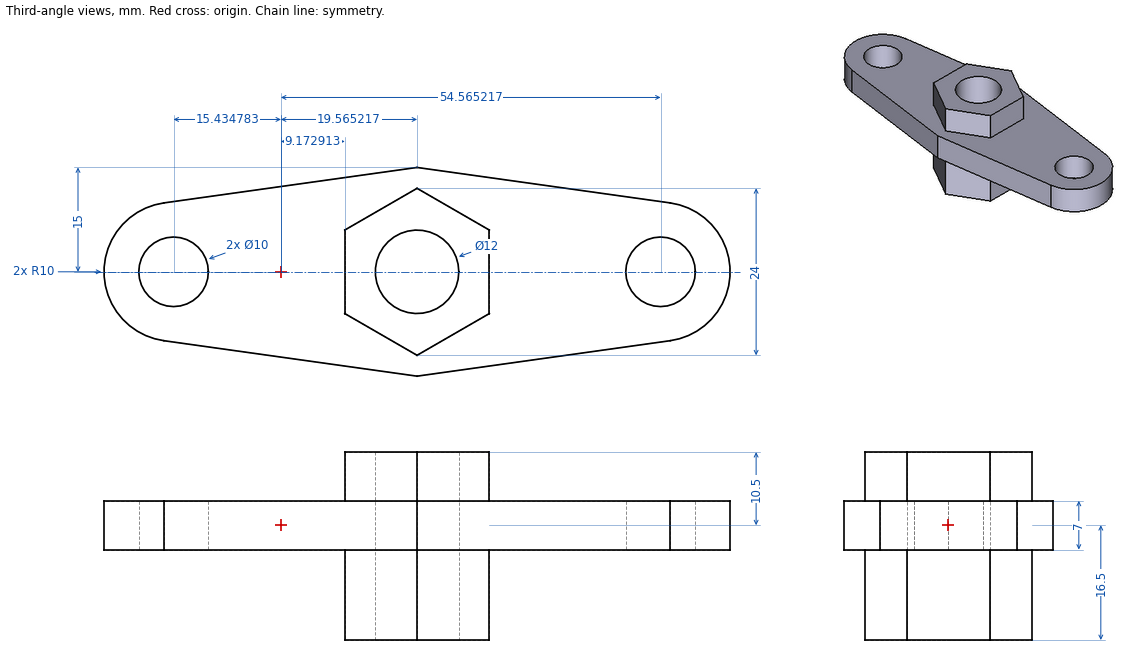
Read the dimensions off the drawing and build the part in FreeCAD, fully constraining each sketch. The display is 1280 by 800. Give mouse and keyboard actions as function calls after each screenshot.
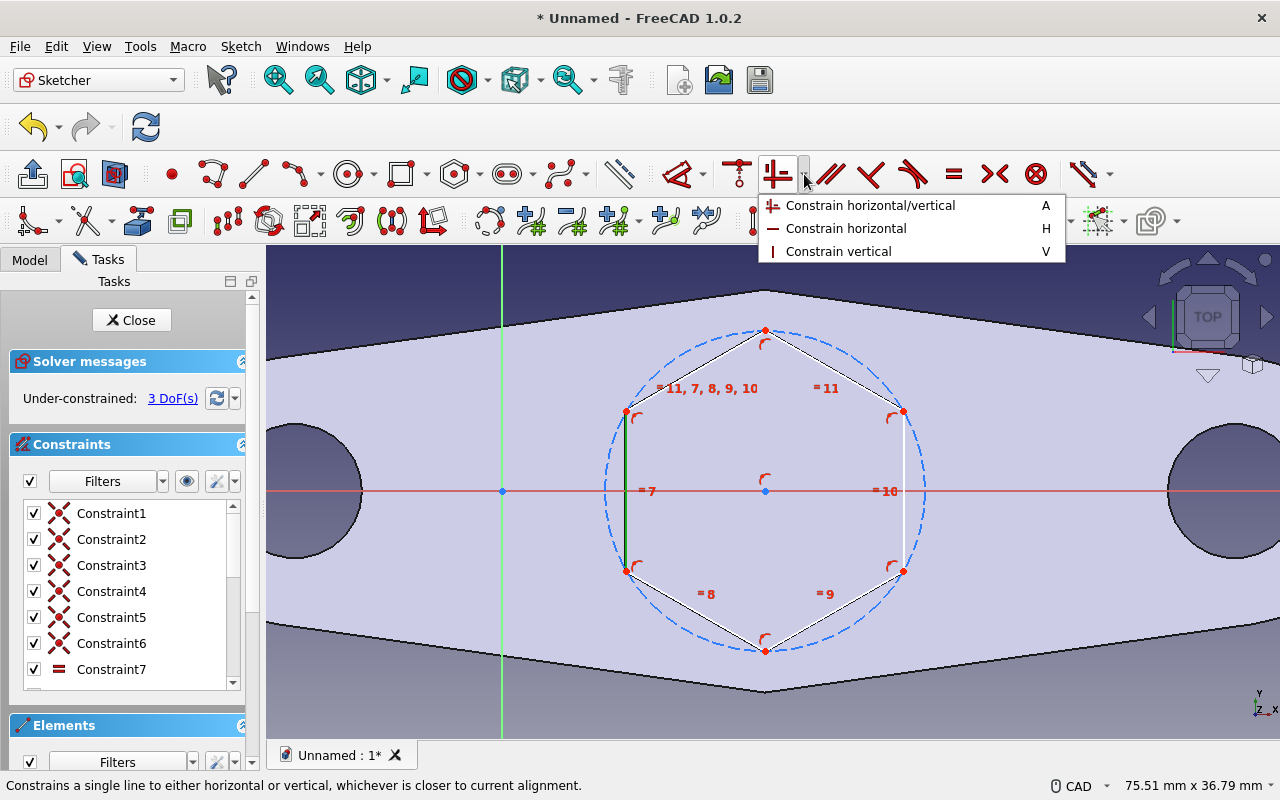
click(912, 252)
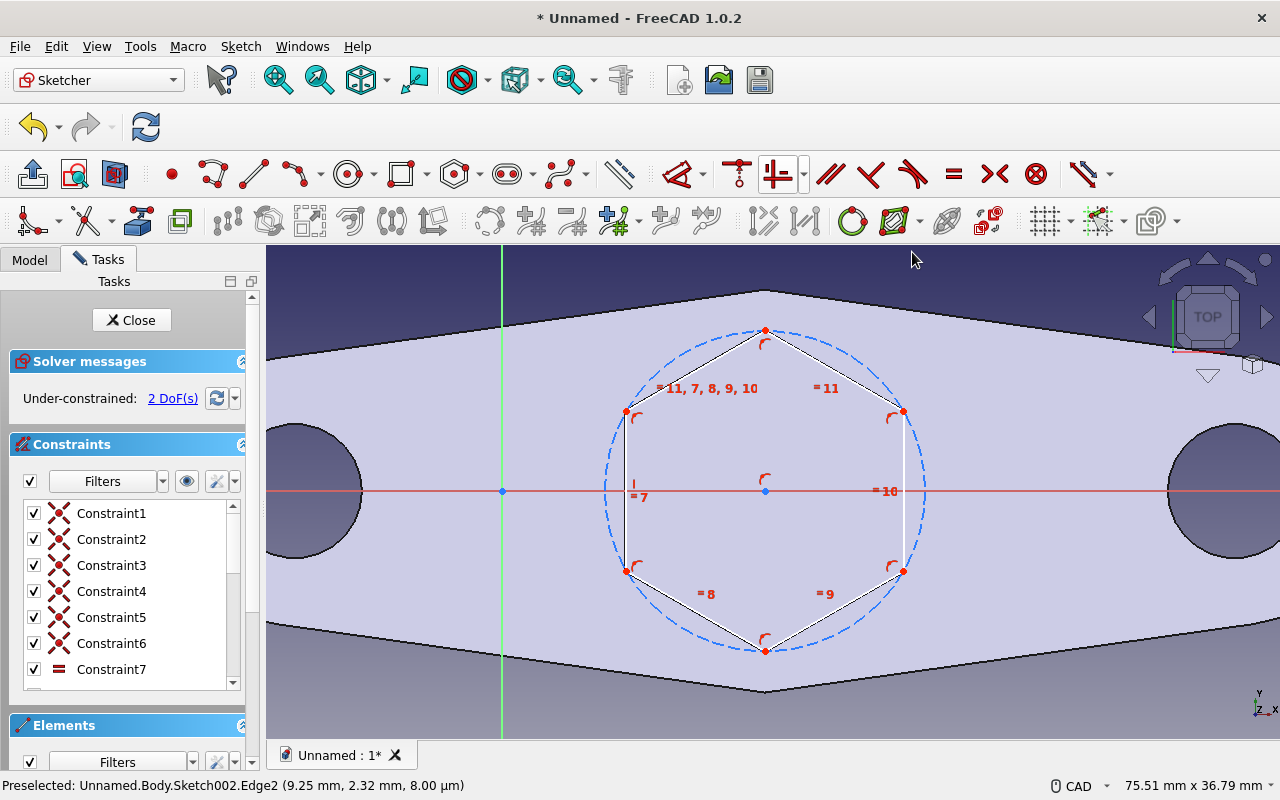
click(676, 174)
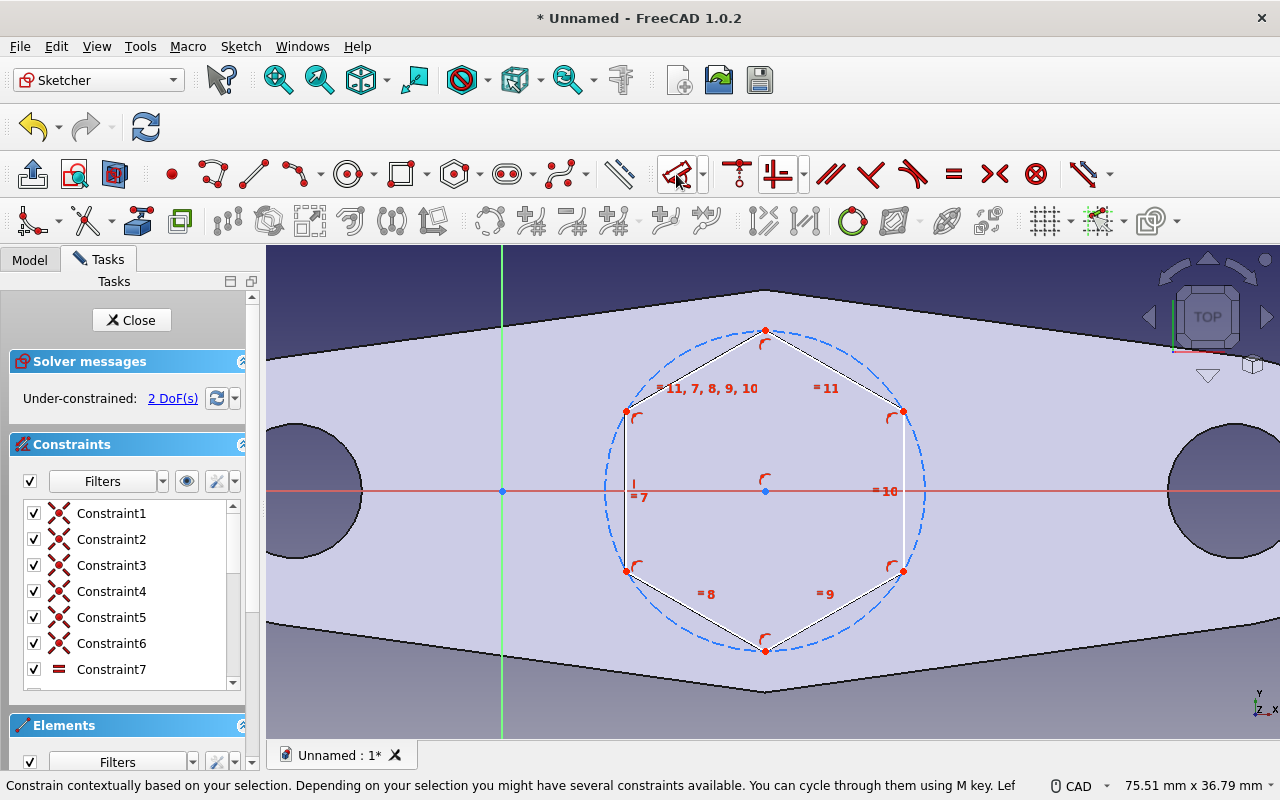
click(765, 651)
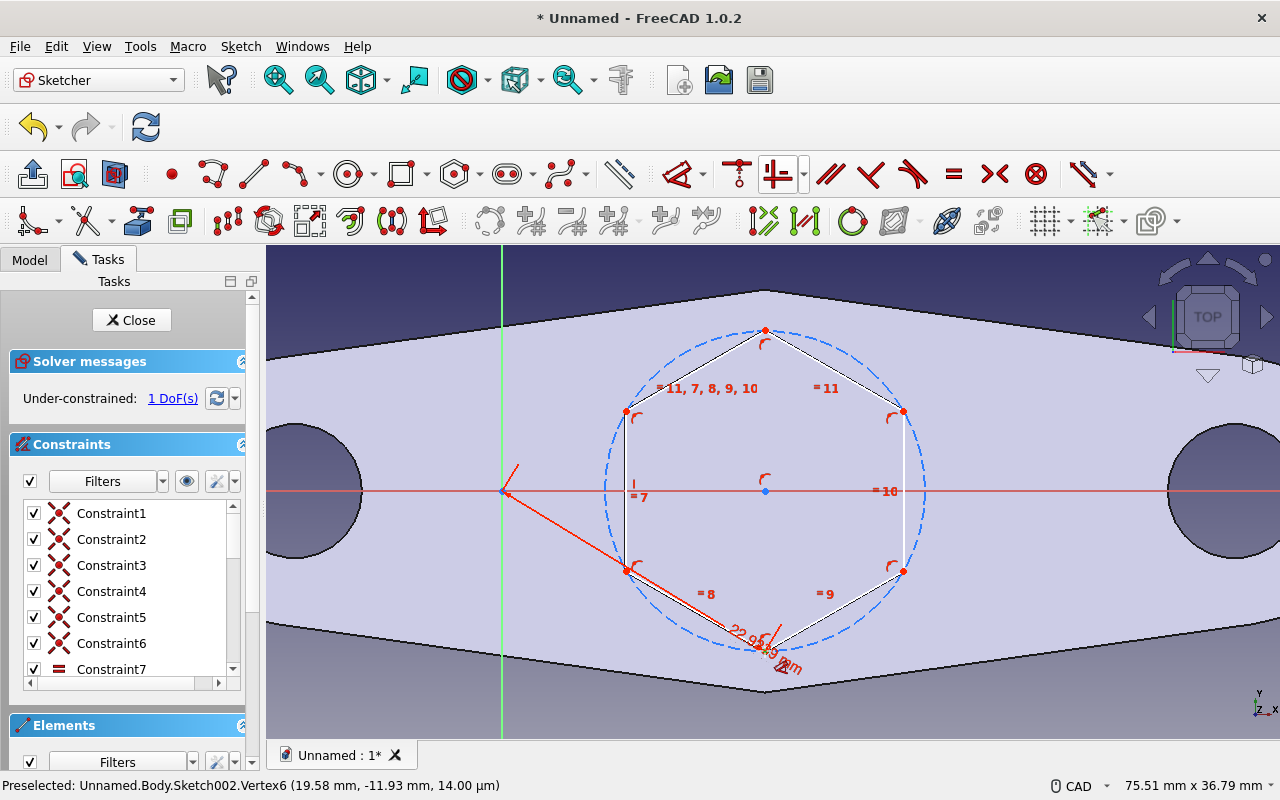
click(765, 331)
click(799, 417)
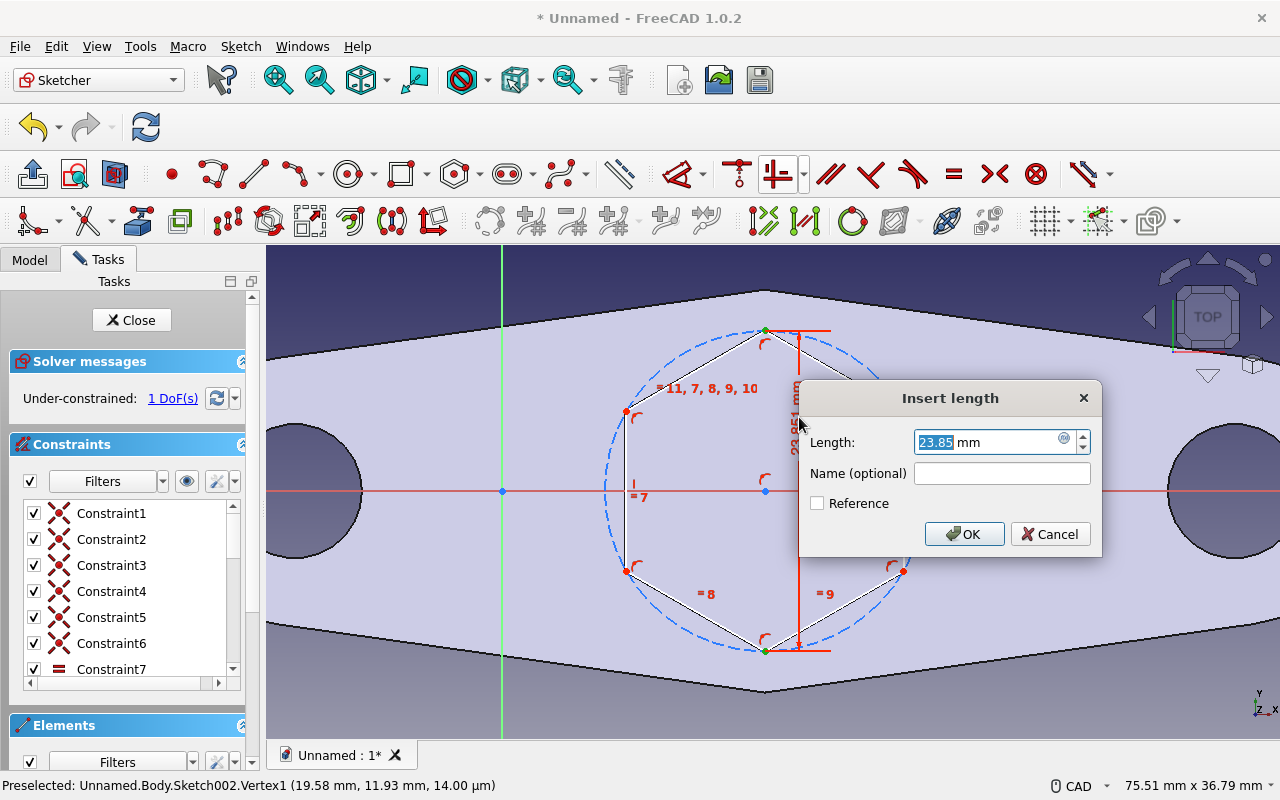
text(24)
key(Return)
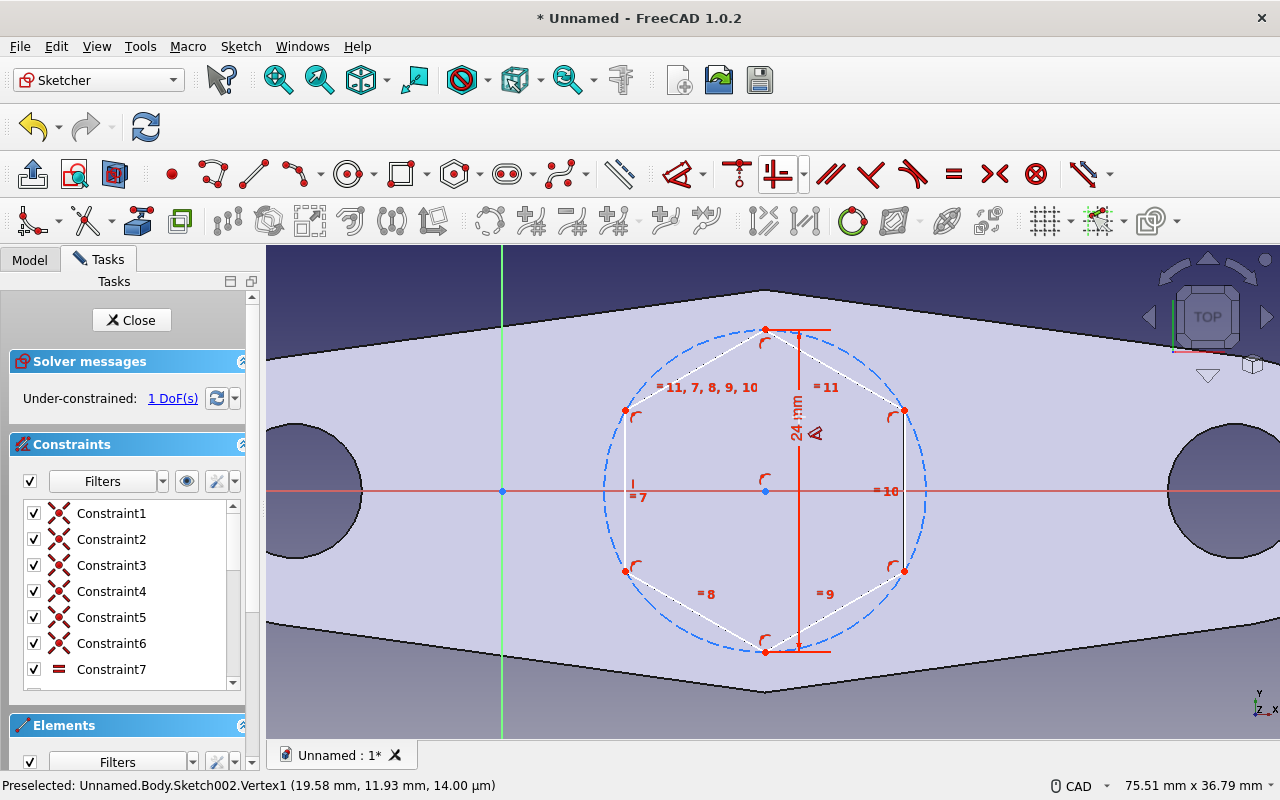
click(625, 411)
click(564, 377)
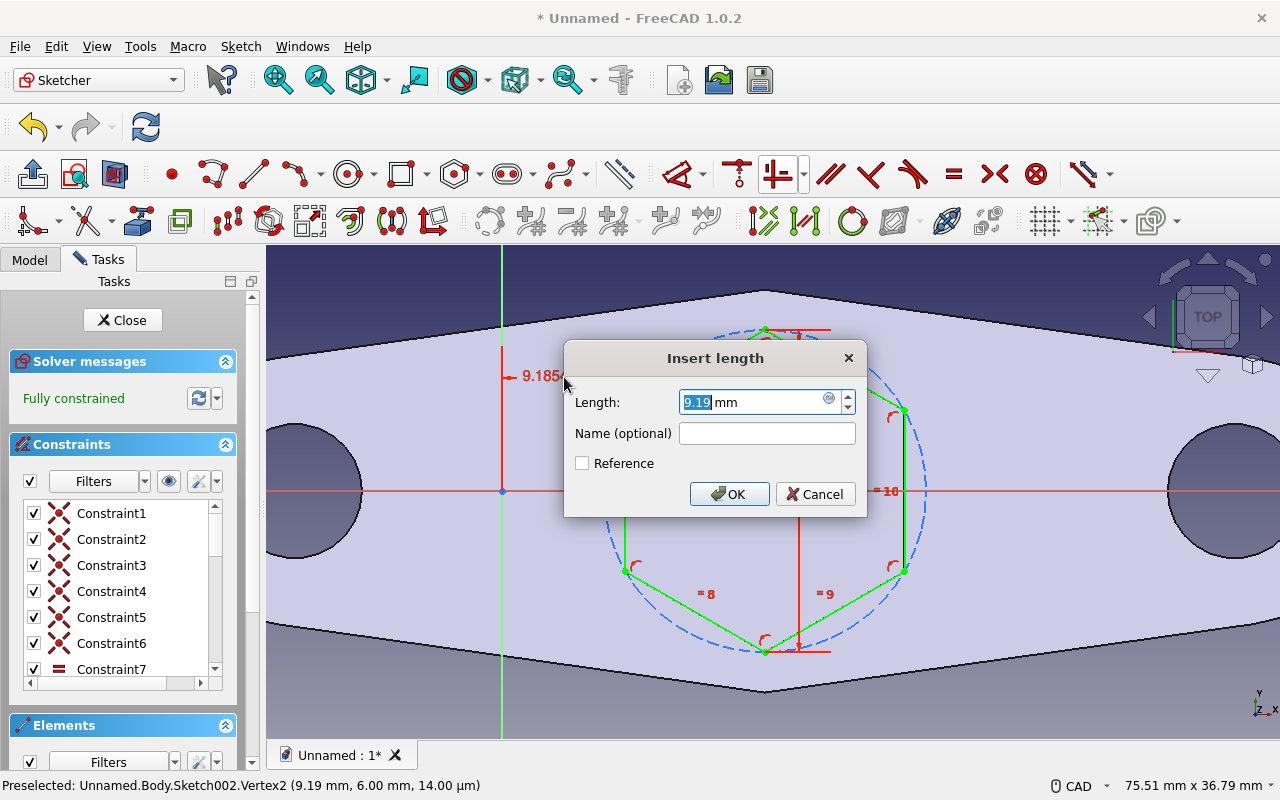
text(9.172913)
key(Return)
key(Escape)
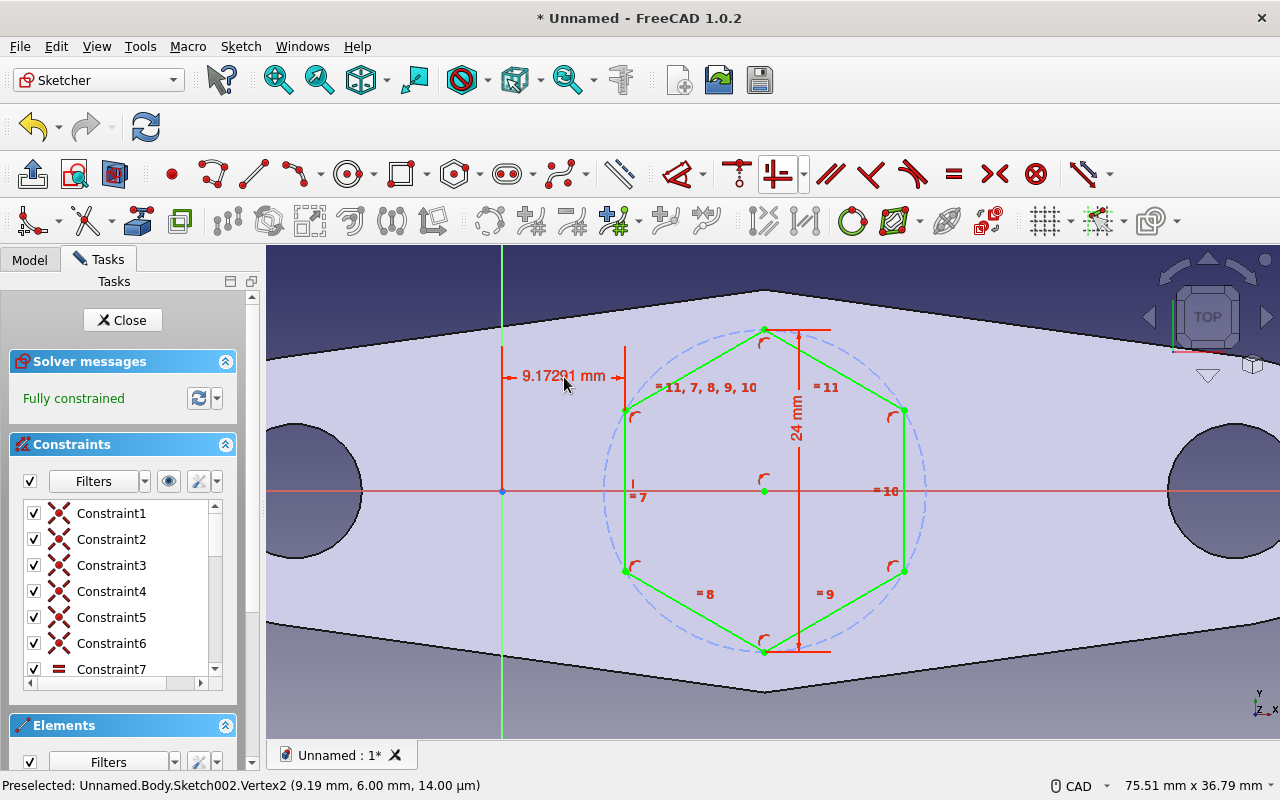
click(123, 320)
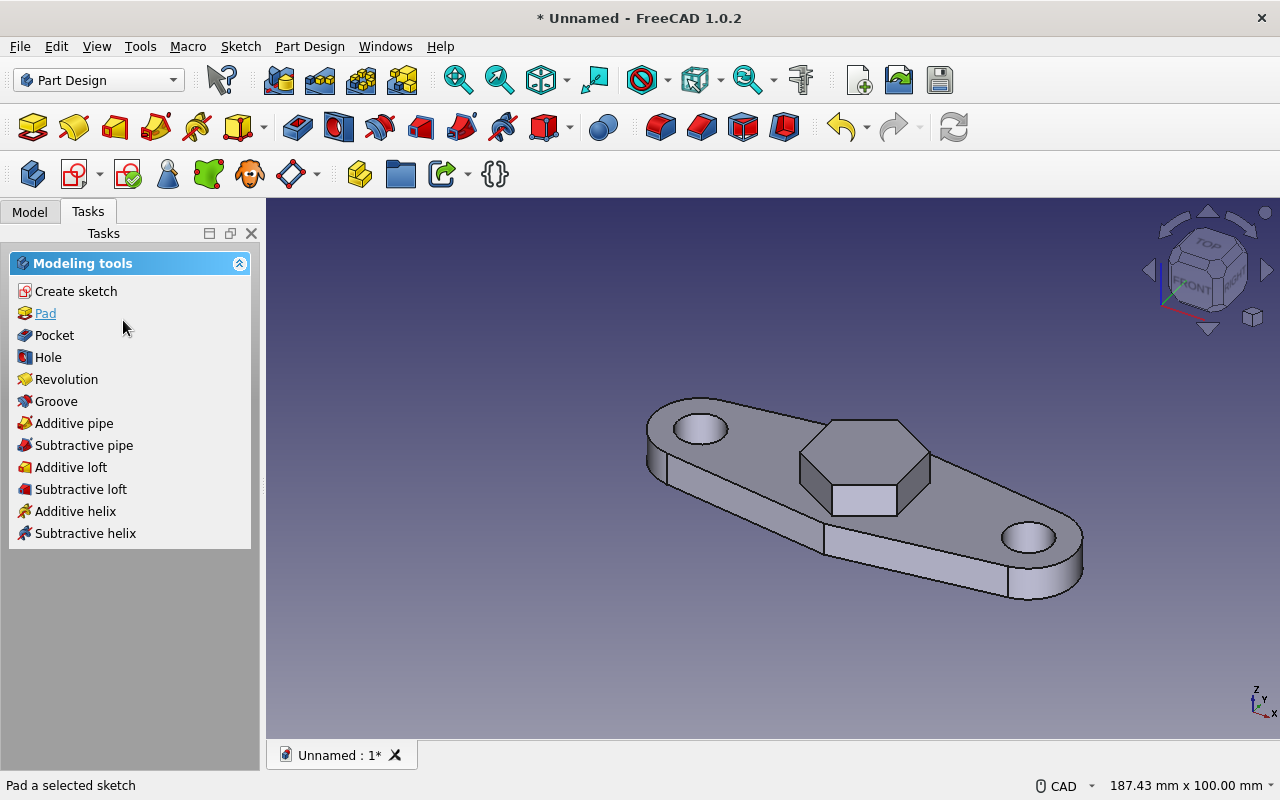
click(33, 128)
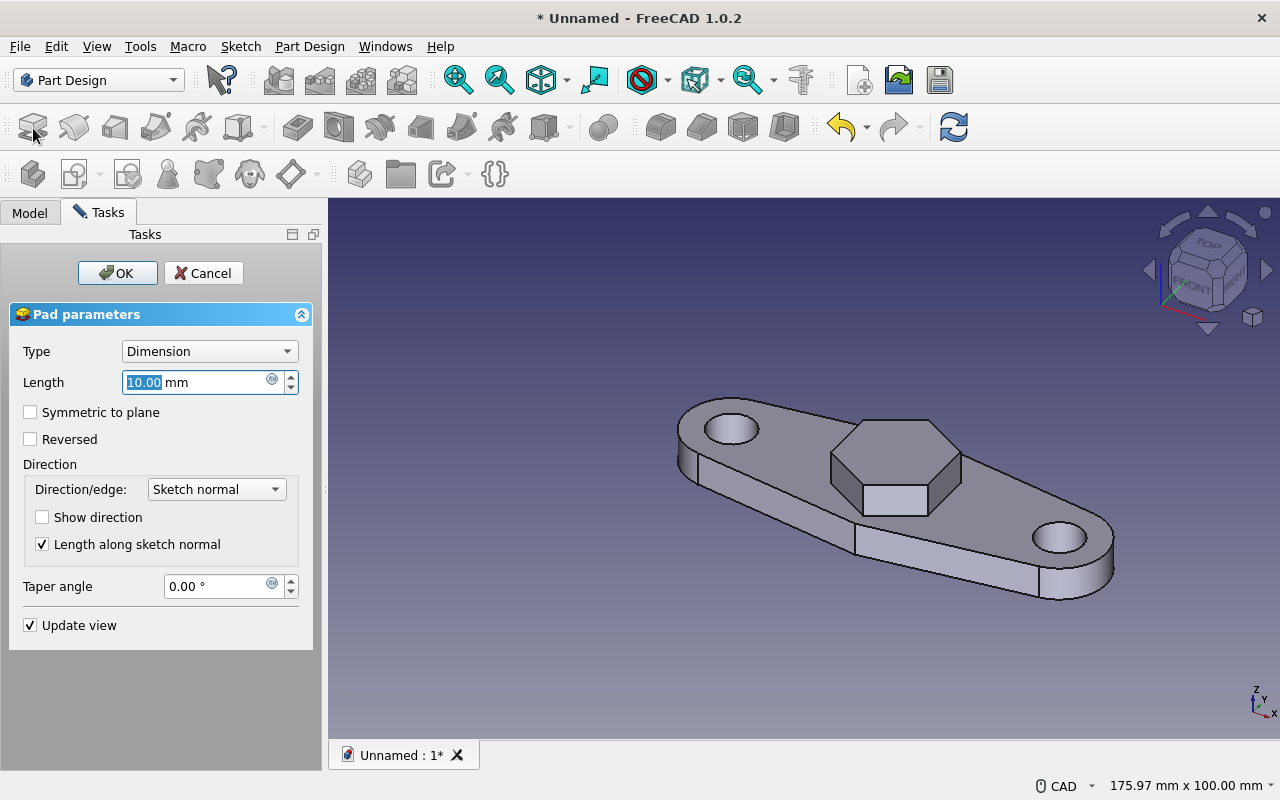
text(16.5)
key(Tab)